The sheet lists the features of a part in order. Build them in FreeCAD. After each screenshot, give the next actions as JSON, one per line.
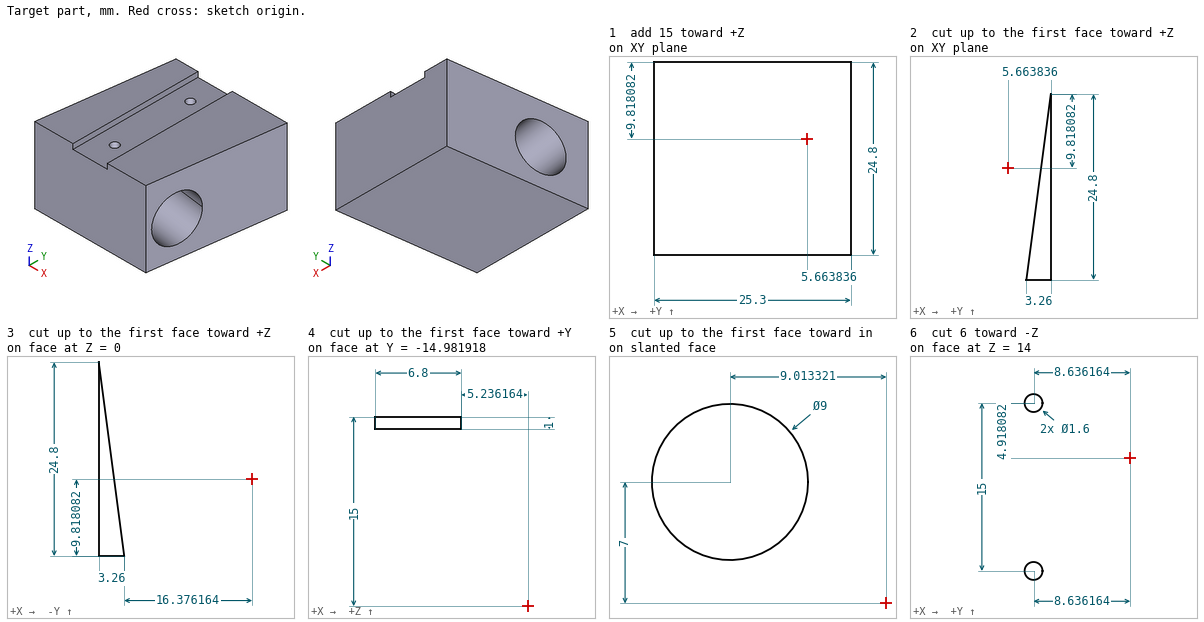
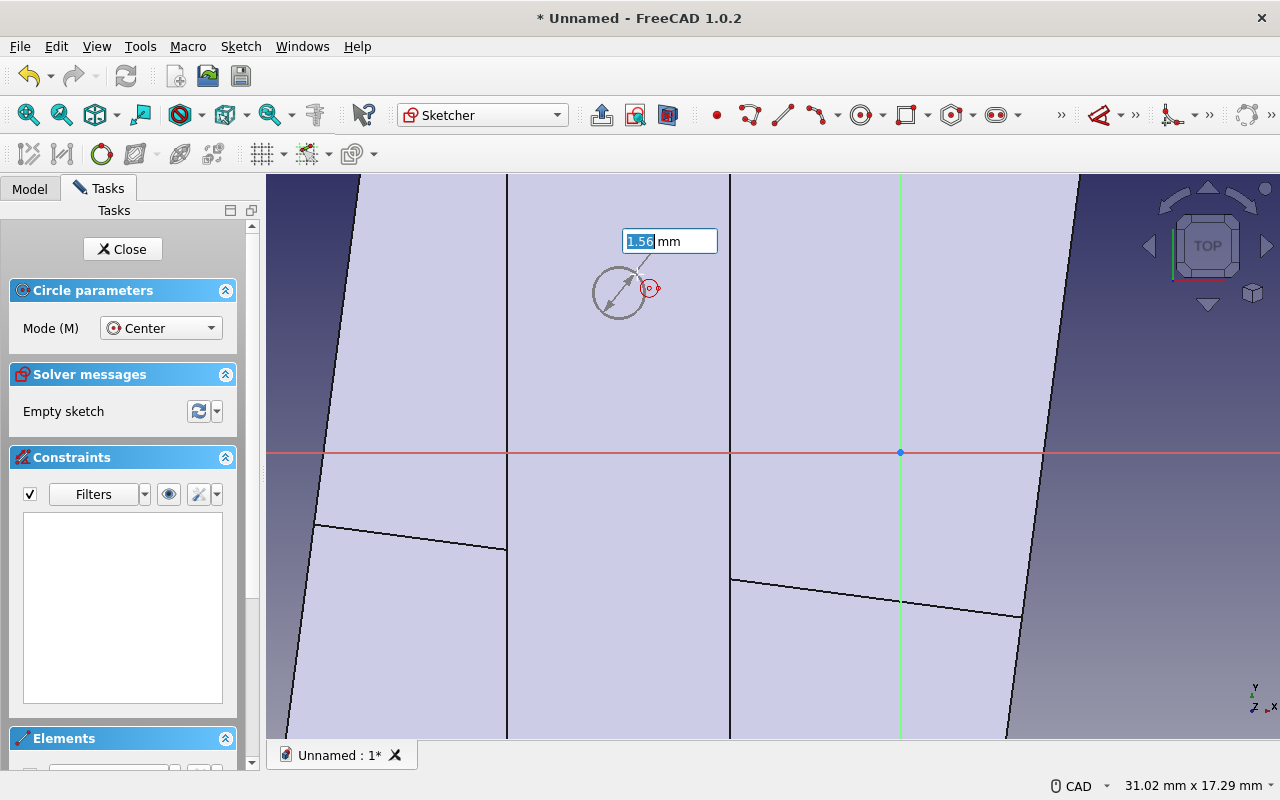
{"action": "type", "text": "1.6"}
{"action": "key", "text": "Return"}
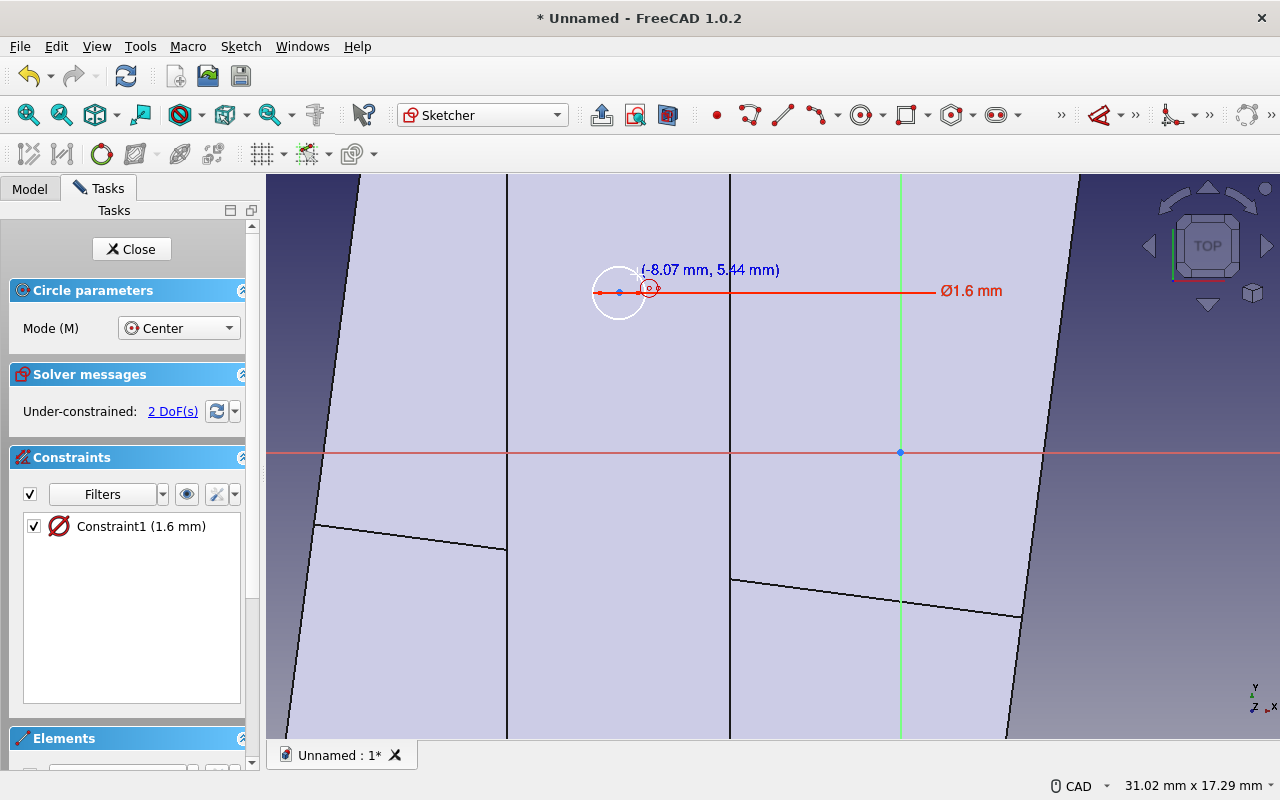
{"action": "scroll", "coordinate": [619, 292], "scroll_direction": "down", "scroll_amount": 2}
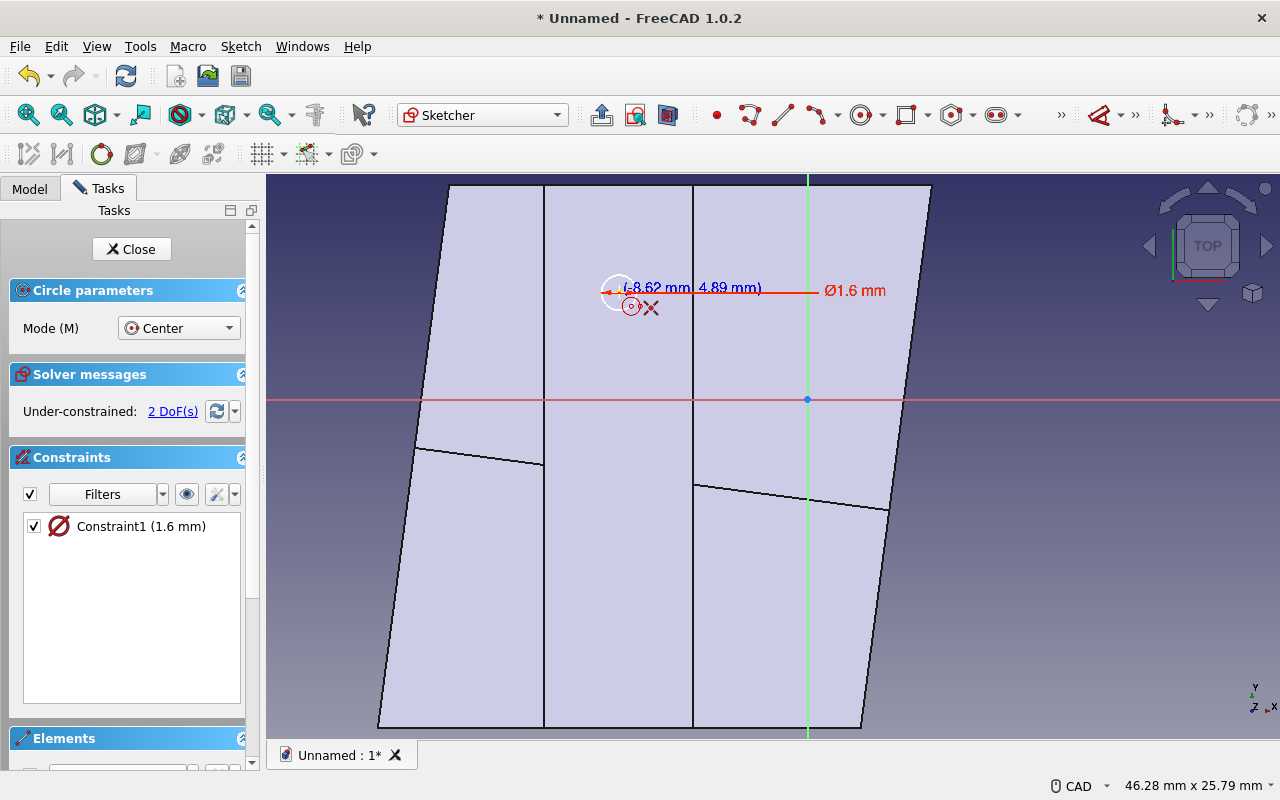
{"action": "scroll", "coordinate": [619, 621], "scroll_direction": "up", "scroll_amount": 2}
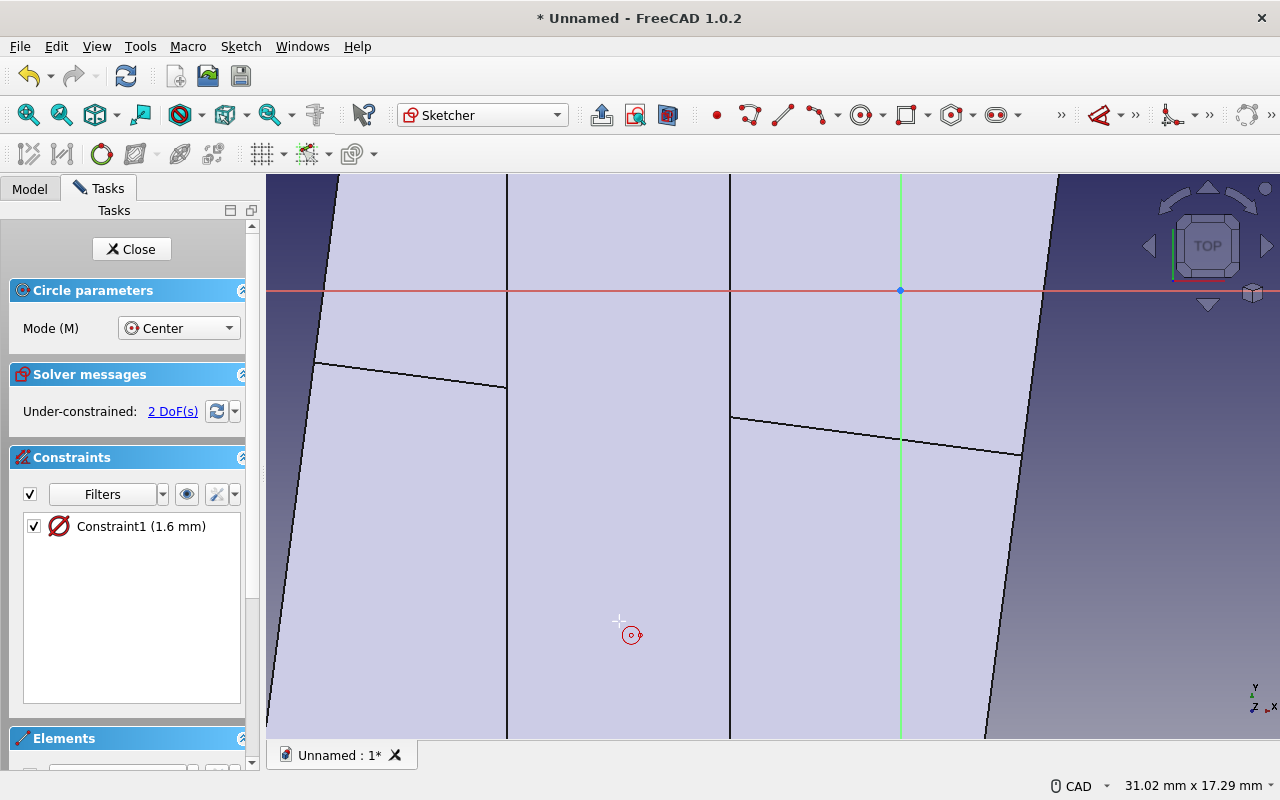
{"action": "left_click", "coordinate": [619, 620]}
{"action": "mouse_move", "coordinate": [637, 602]}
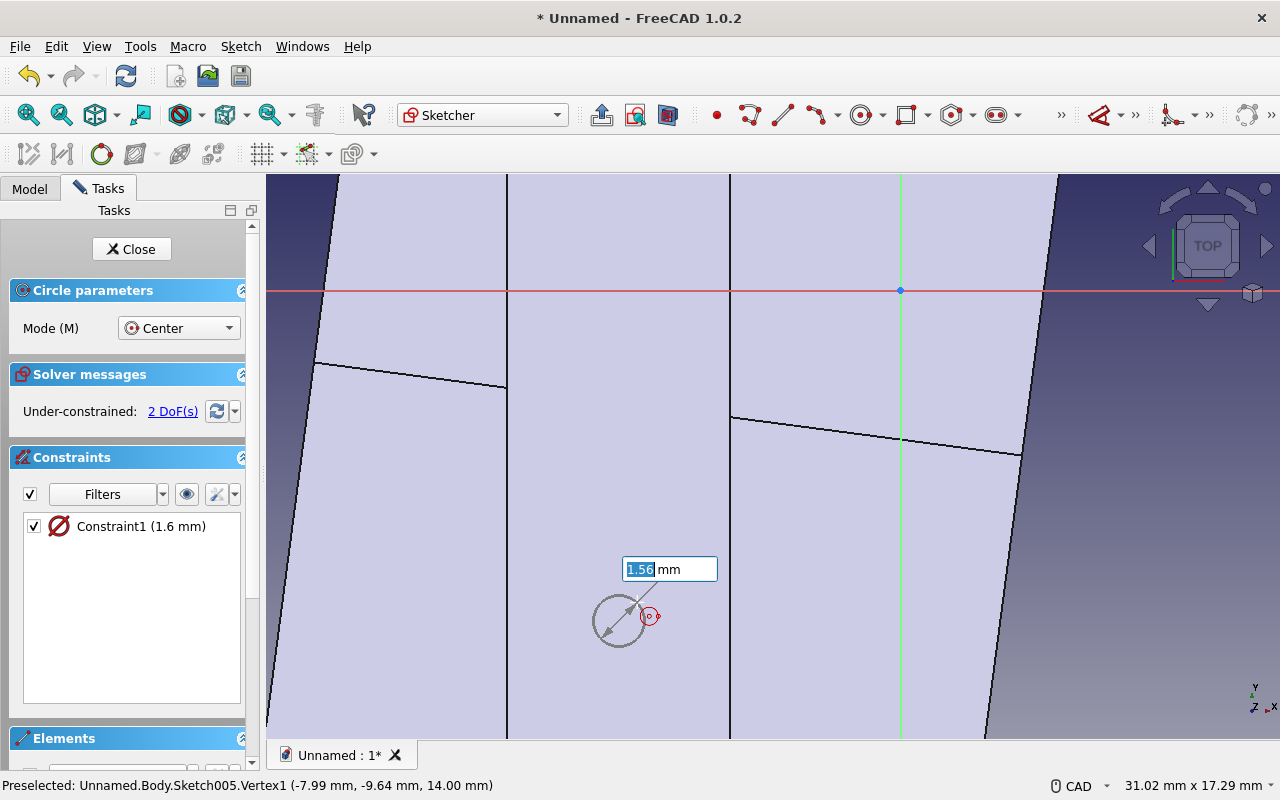
{"action": "type", "text": "1.6"}
{"action": "key", "text": "Return"}
{"action": "key", "text": "Escape"}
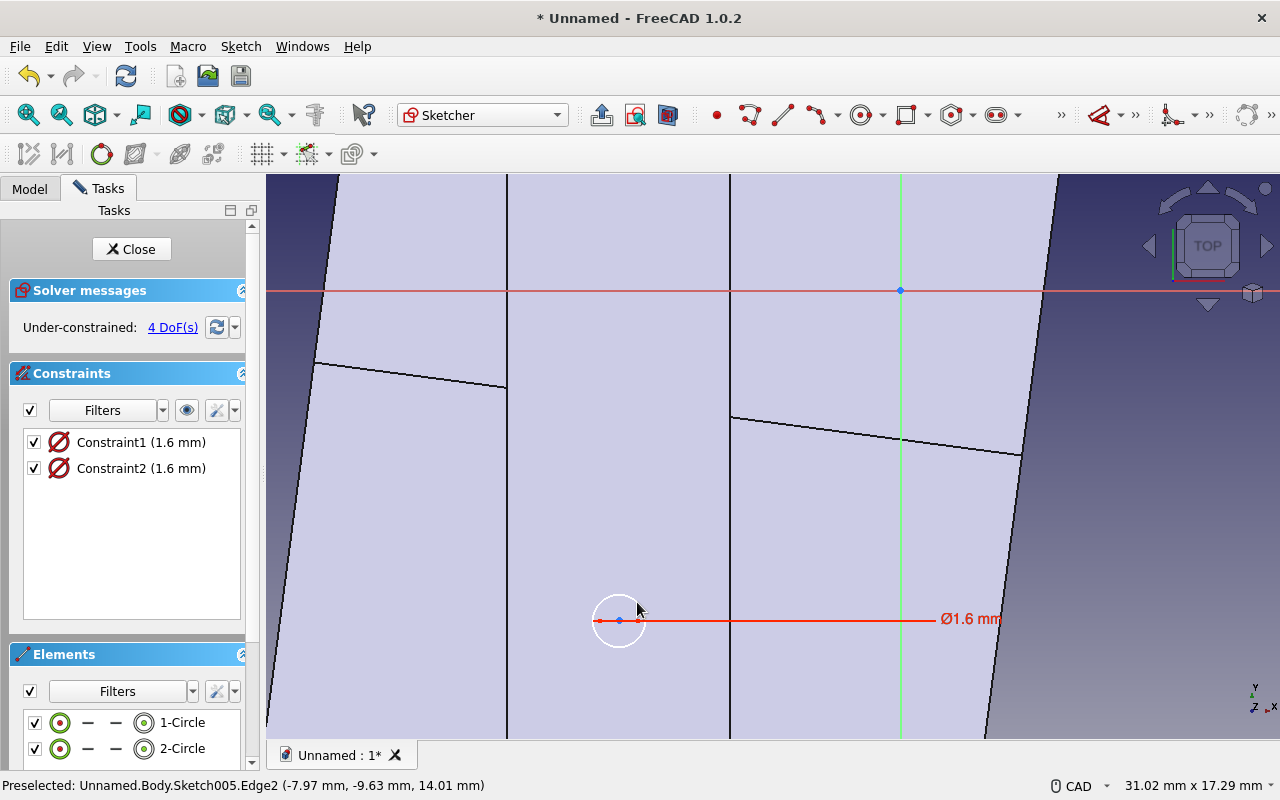
{"action": "left_click", "coordinate": [1098, 116]}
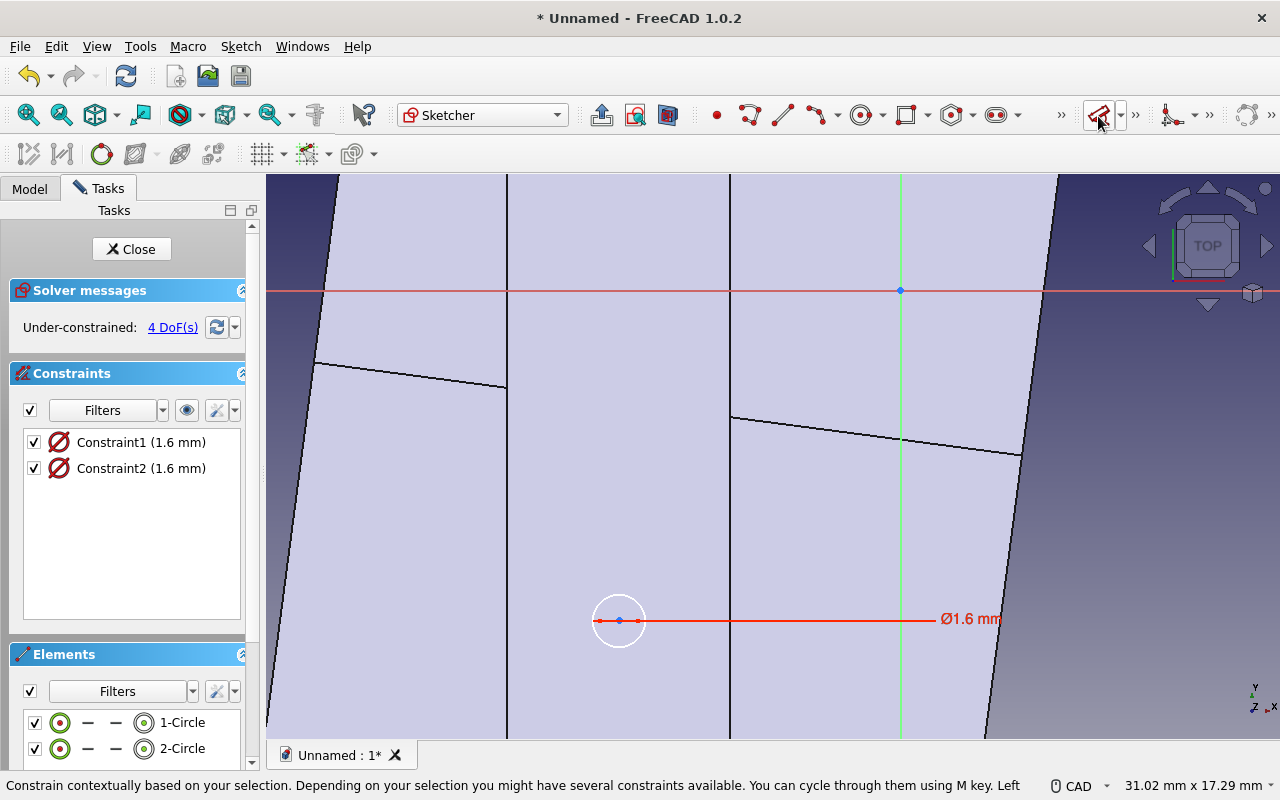
{"action": "scroll", "coordinate": [619, 622], "scroll_direction": "down", "scroll_amount": 2}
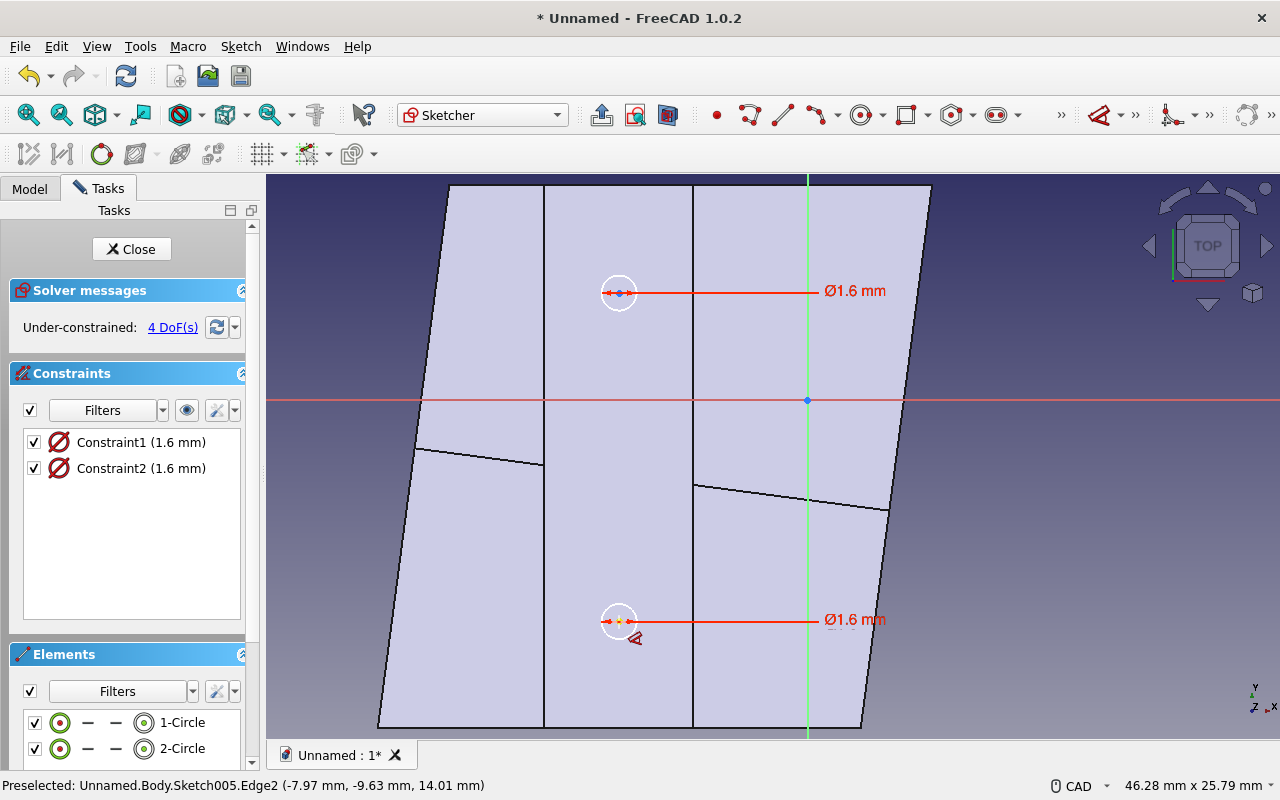
{"action": "left_click", "coordinate": [619, 293]}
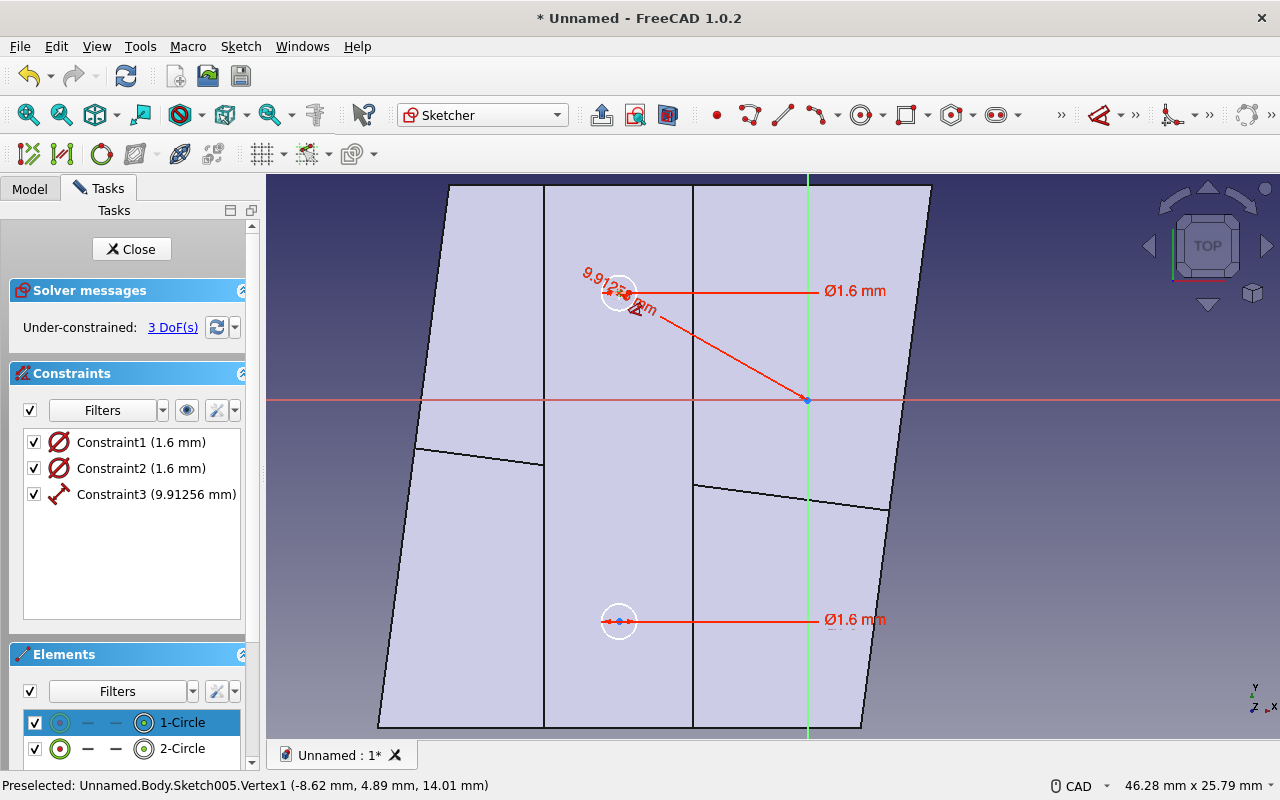
{"action": "left_click", "coordinate": [619, 622]}
{"action": "left_click", "coordinate": [585, 457]}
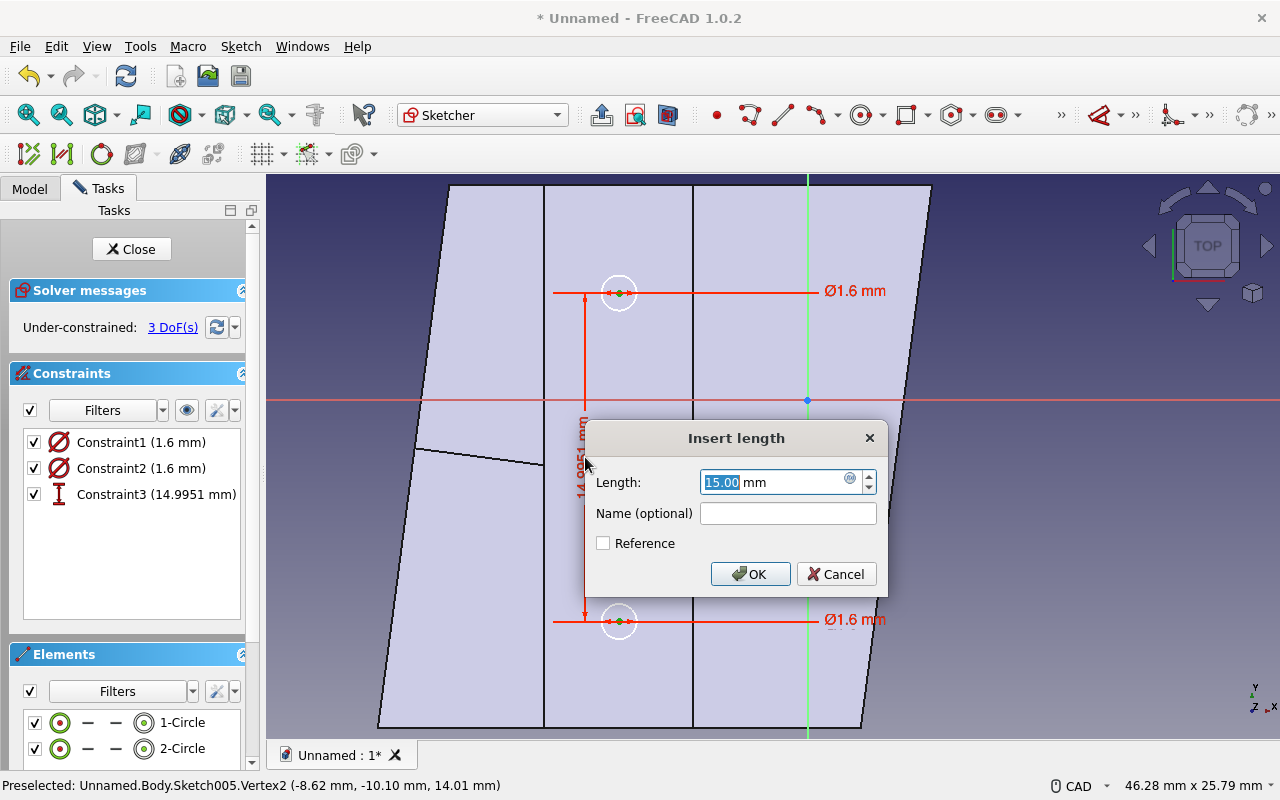
{"action": "type", "text": "15"}
{"action": "key", "text": "Return"}